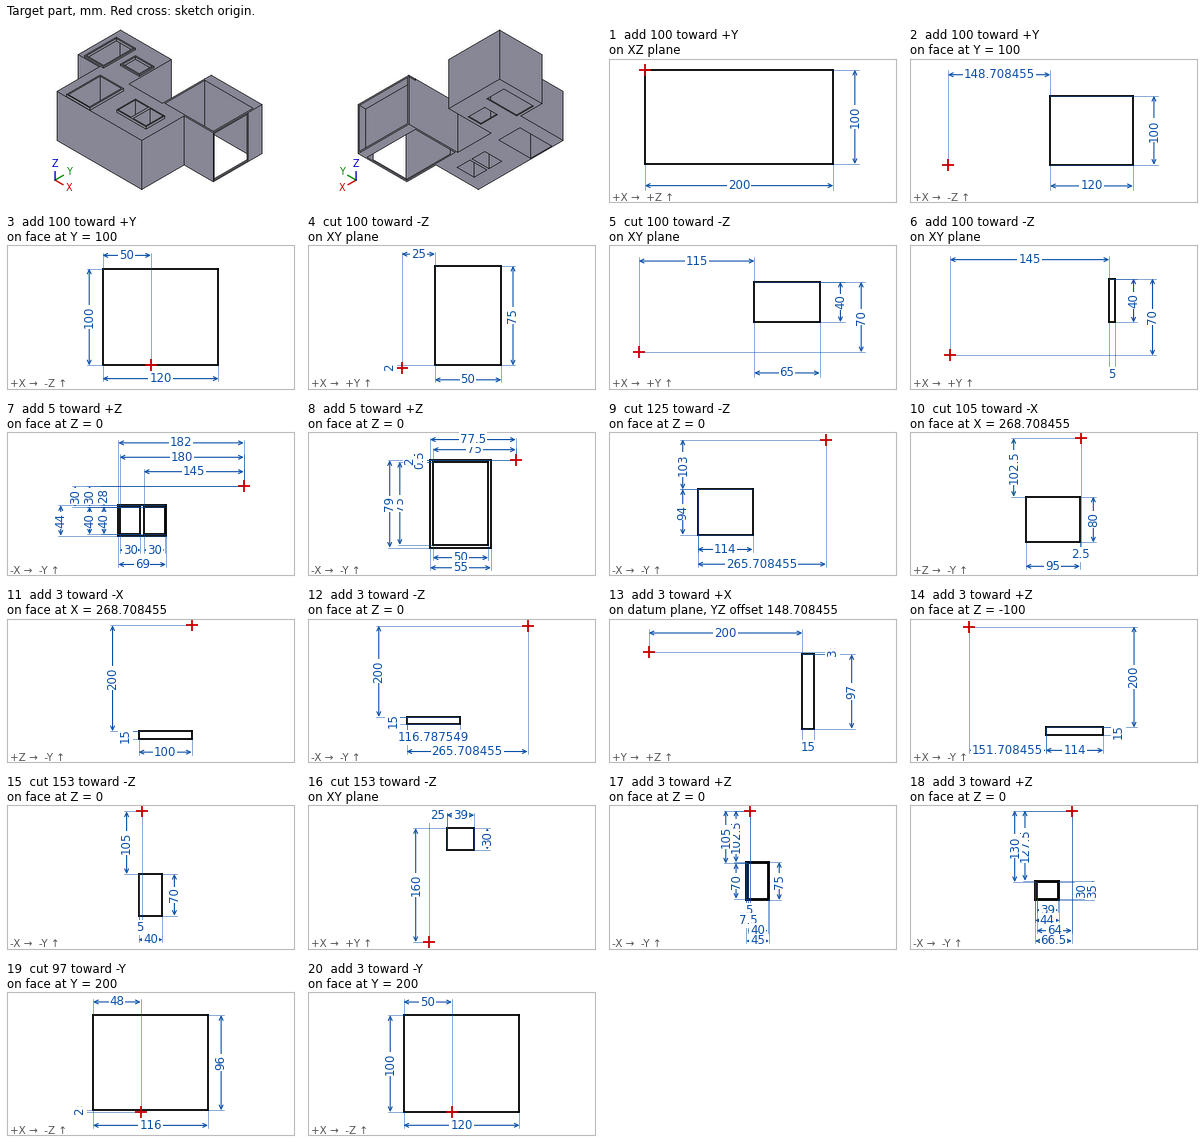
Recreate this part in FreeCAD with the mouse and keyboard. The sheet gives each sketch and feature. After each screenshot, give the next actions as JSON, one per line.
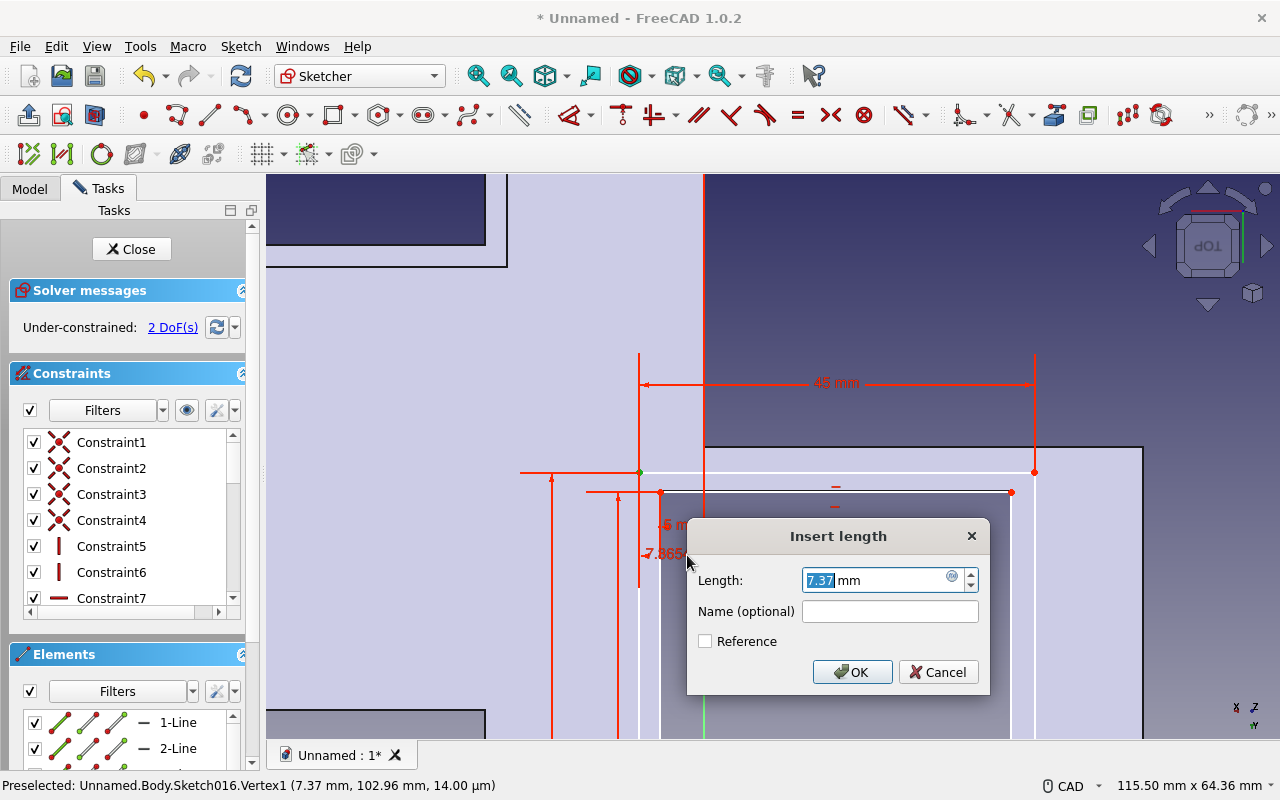
{"action": "type", "text": "7.5"}
{"action": "key", "text": "Return"}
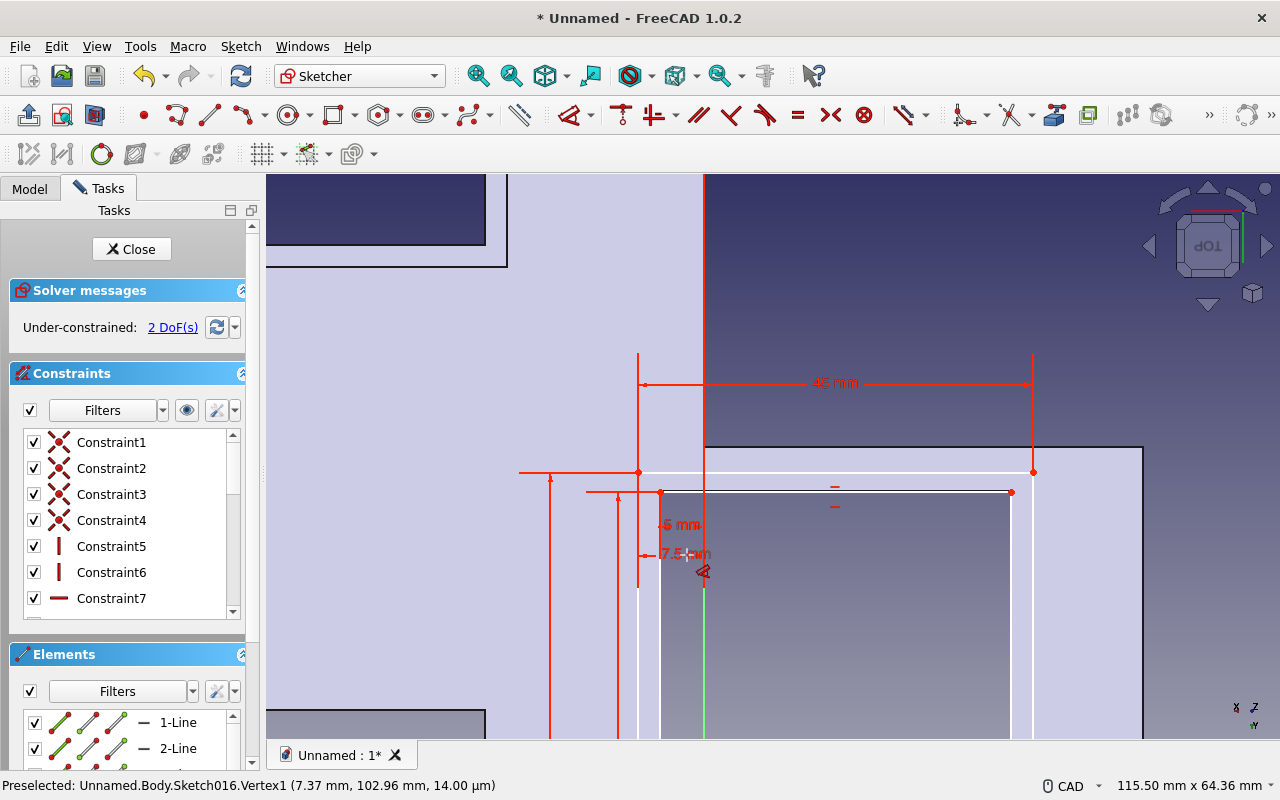
{"action": "left_click", "coordinate": [660, 492]}
{"action": "left_click", "coordinate": [626, 347]}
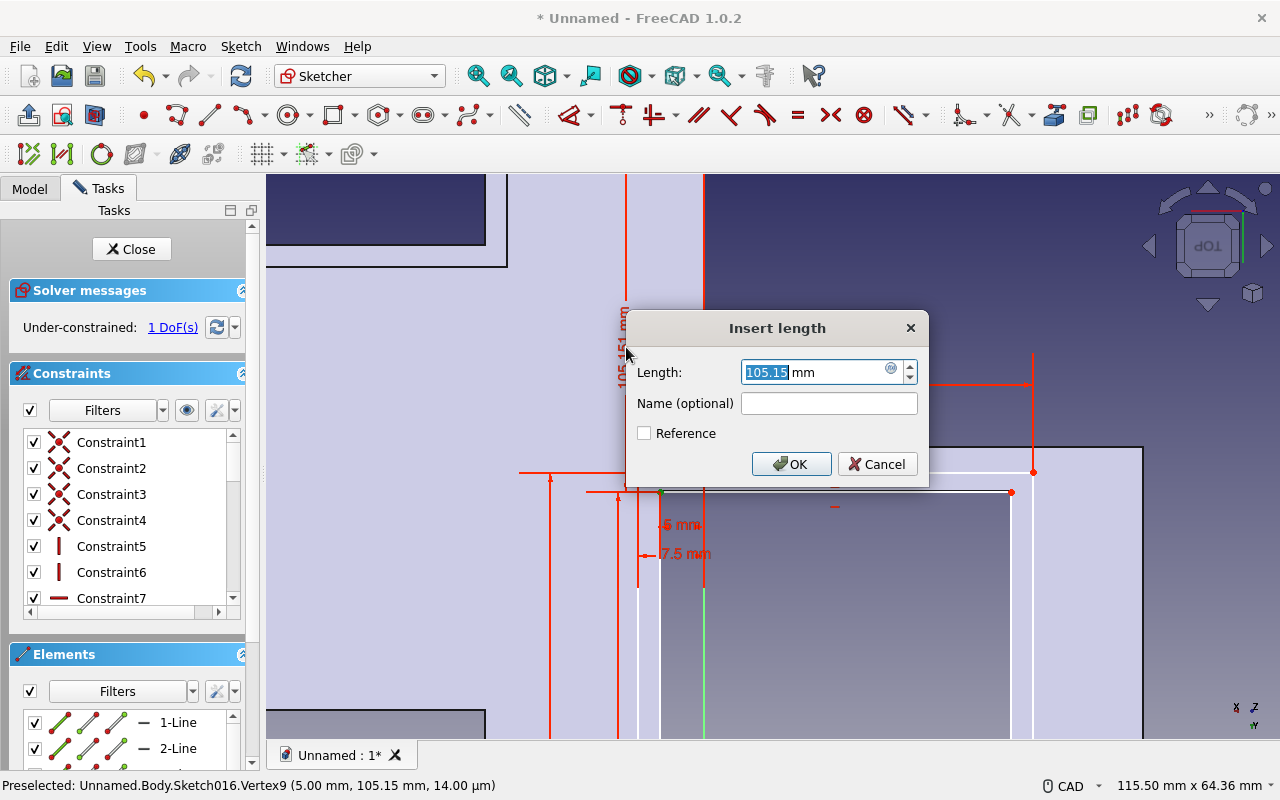
{"action": "type", "text": "105"}
{"action": "key", "text": "Return"}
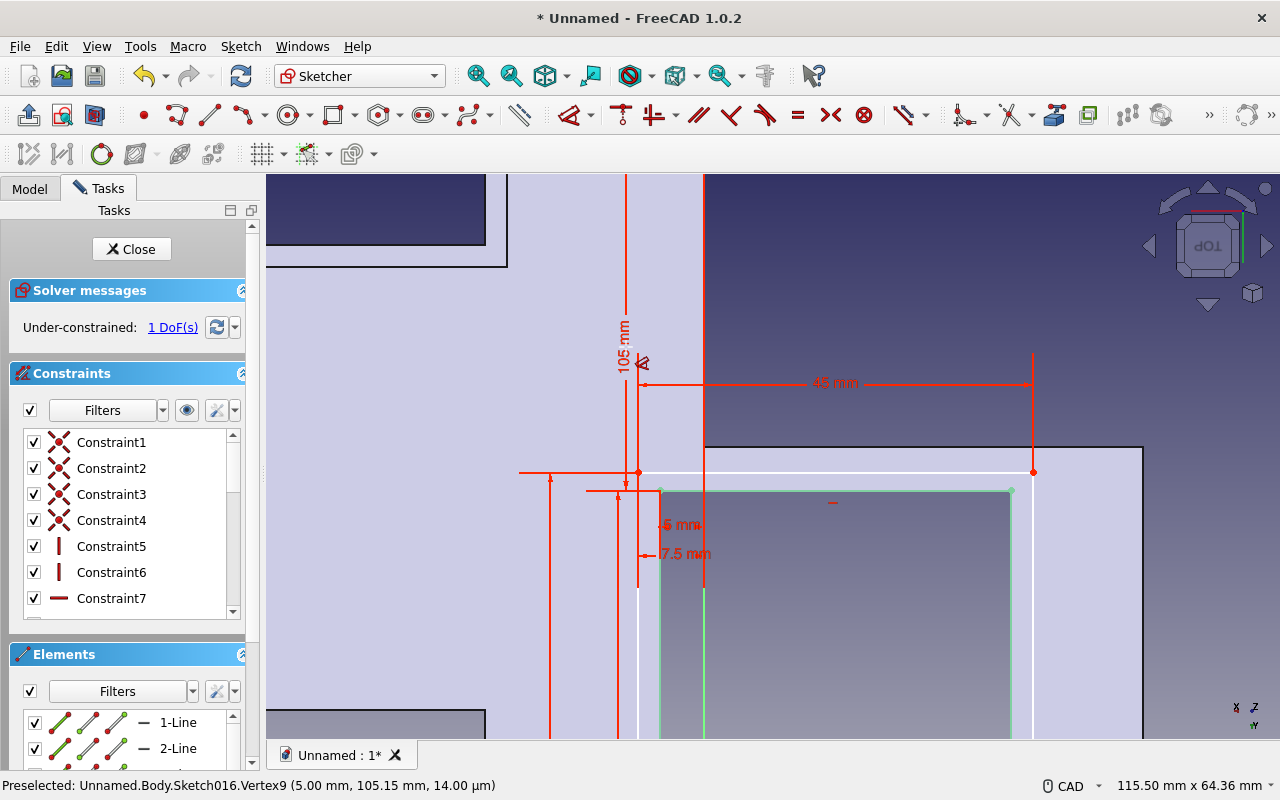
{"action": "left_click", "coordinate": [638, 473]}
{"action": "left_click", "coordinate": [604, 275]}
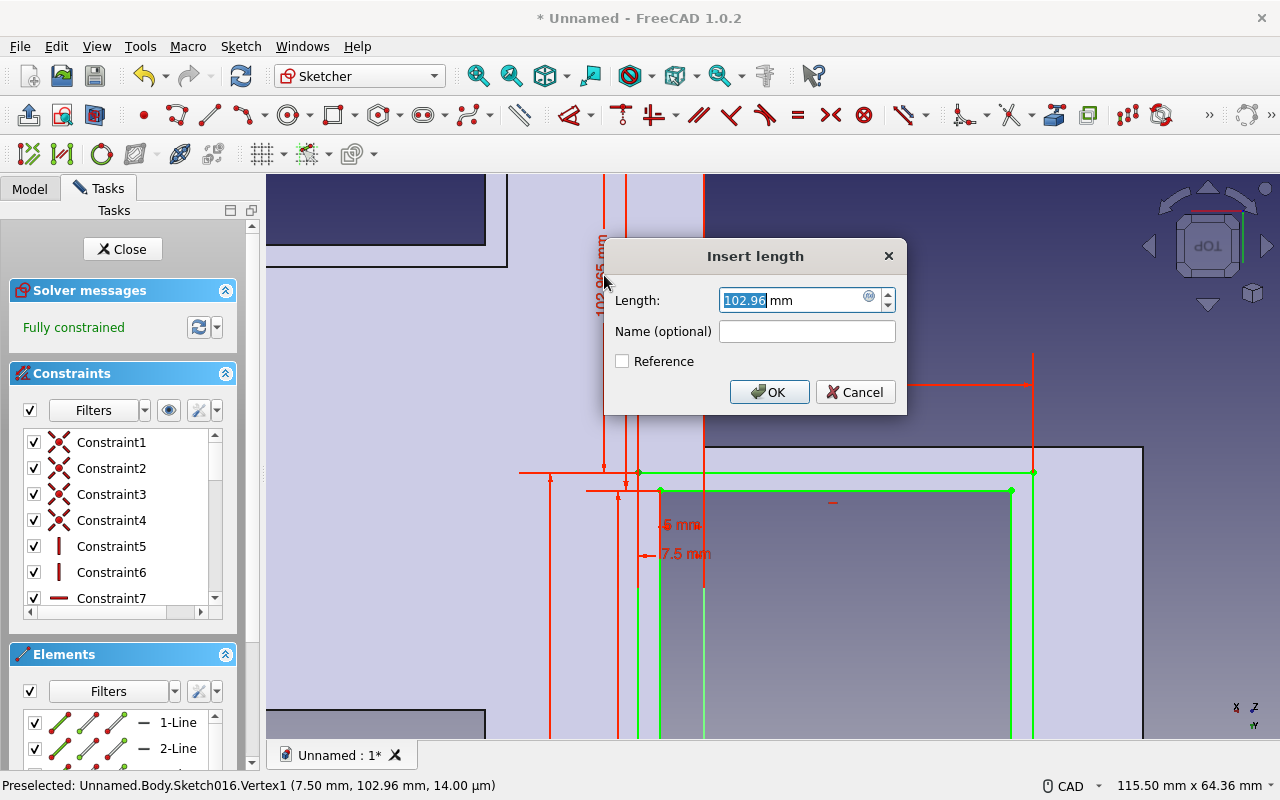
{"action": "type", "text": "102.5"}
{"action": "key", "text": "Return"}
{"action": "key", "text": "Escape"}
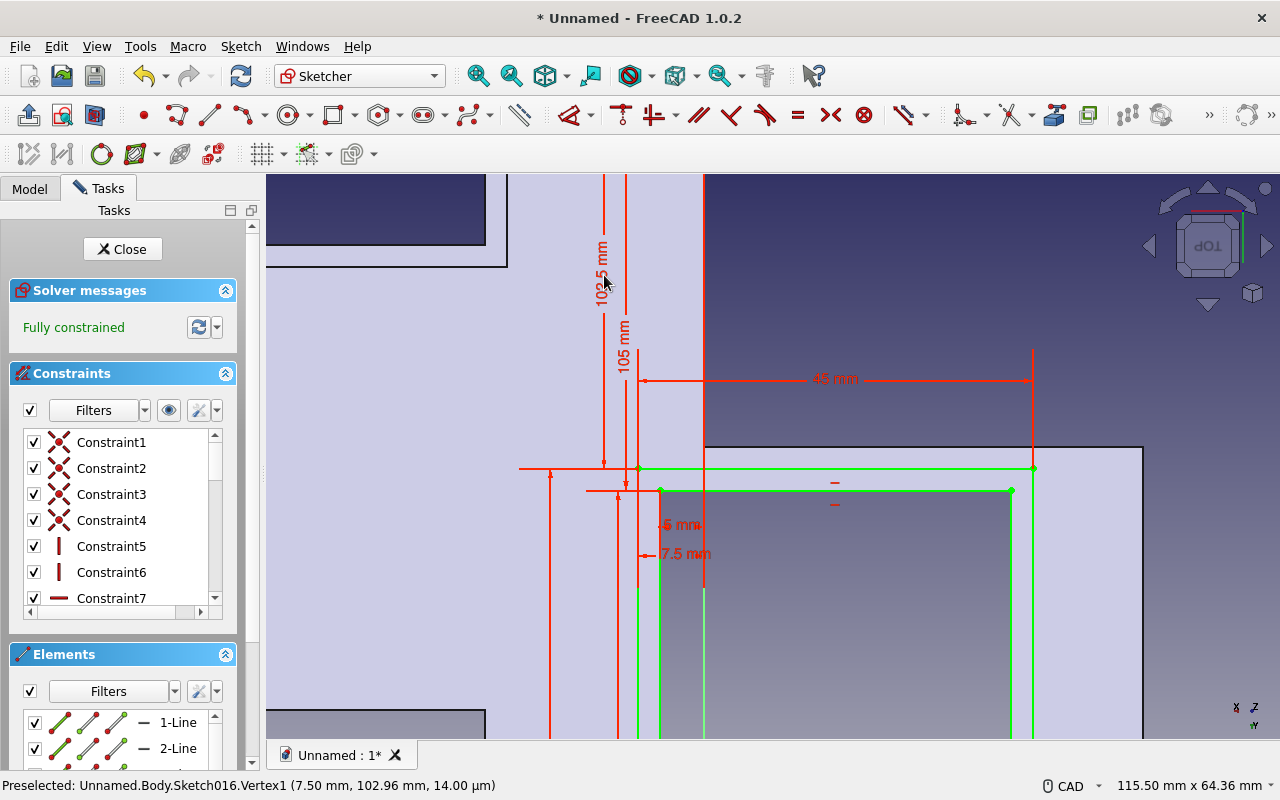
{"action": "left_click", "coordinate": [123, 249]}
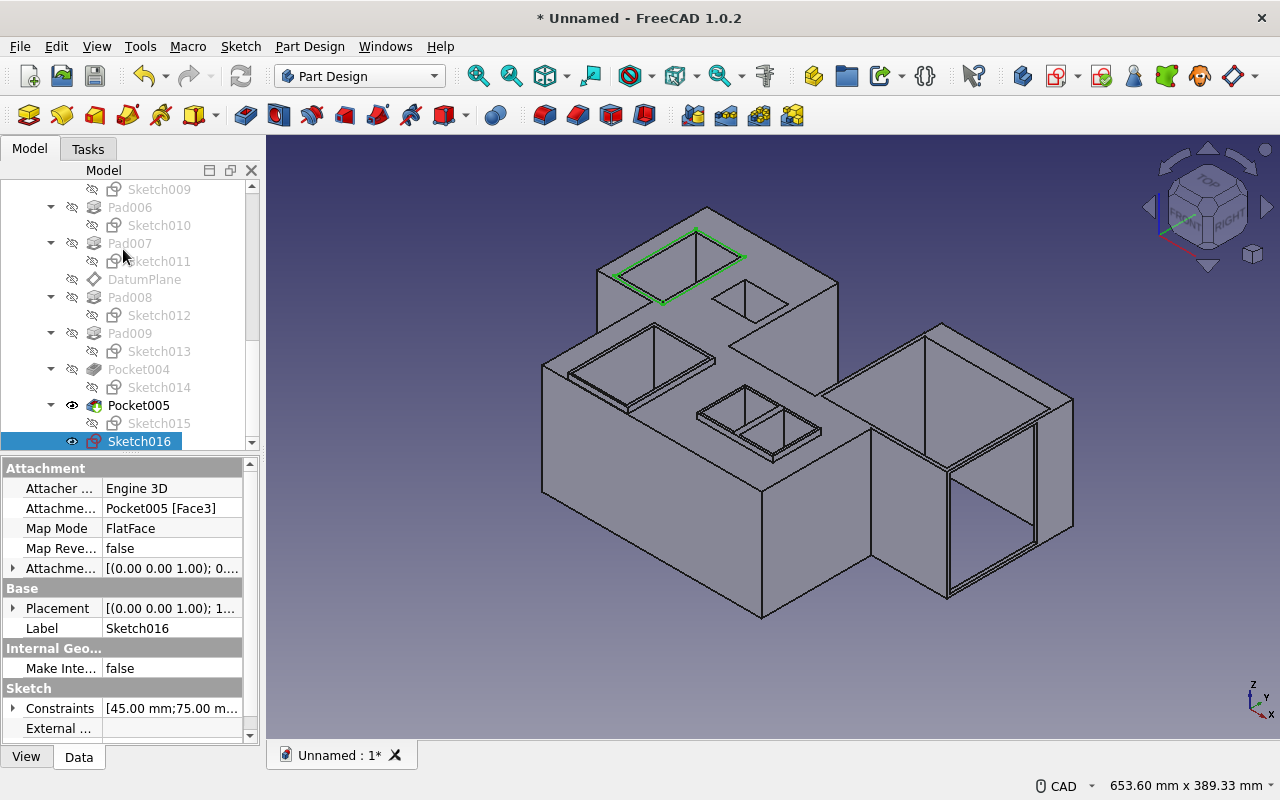
{"action": "left_click", "coordinate": [29, 116]}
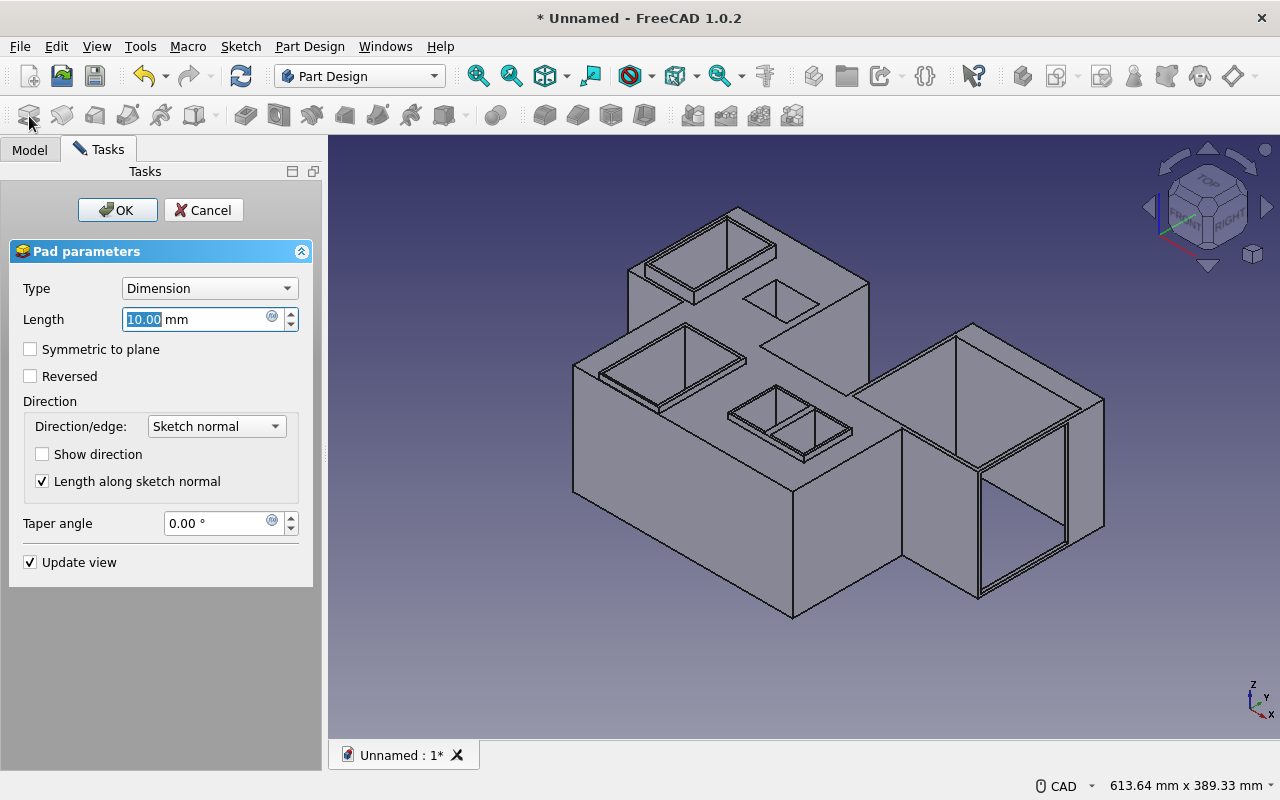
{"action": "type", "text": "3"}
{"action": "key", "text": "Tab"}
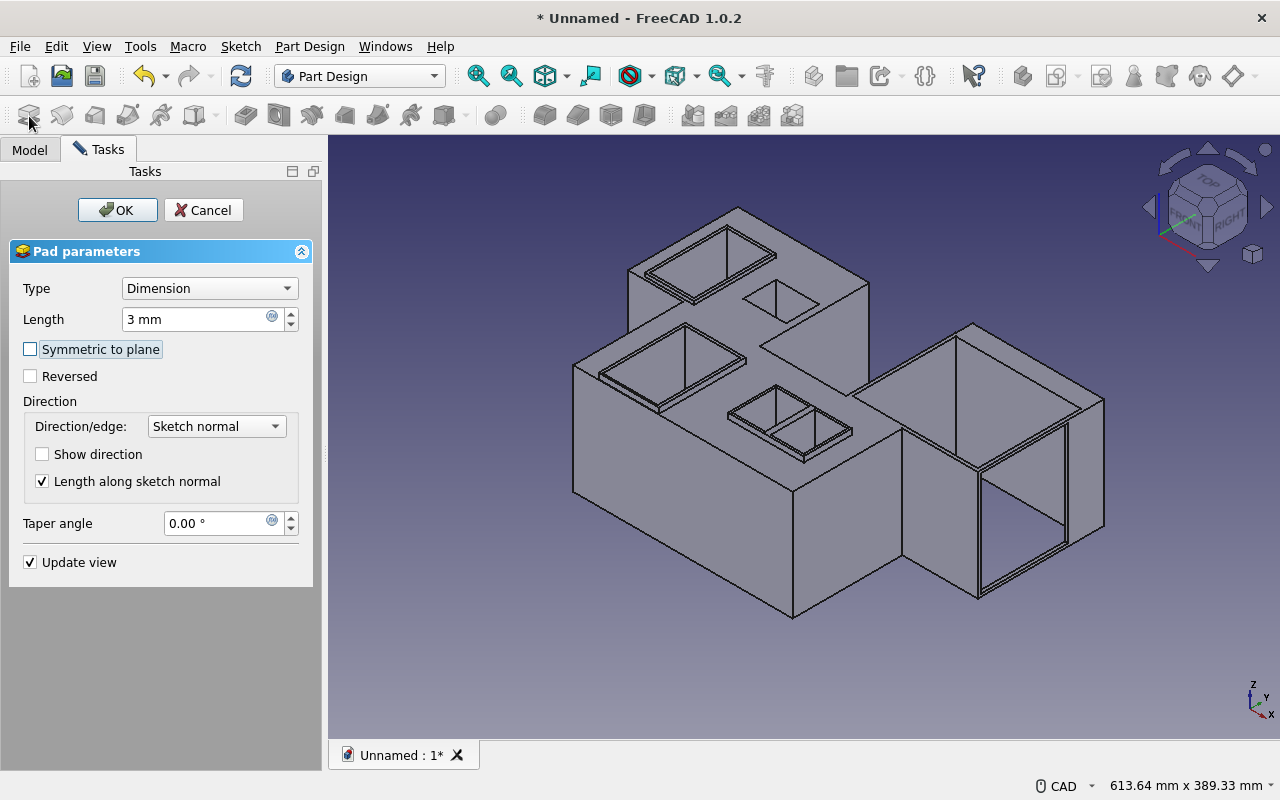
{"action": "left_click", "coordinate": [118, 210]}